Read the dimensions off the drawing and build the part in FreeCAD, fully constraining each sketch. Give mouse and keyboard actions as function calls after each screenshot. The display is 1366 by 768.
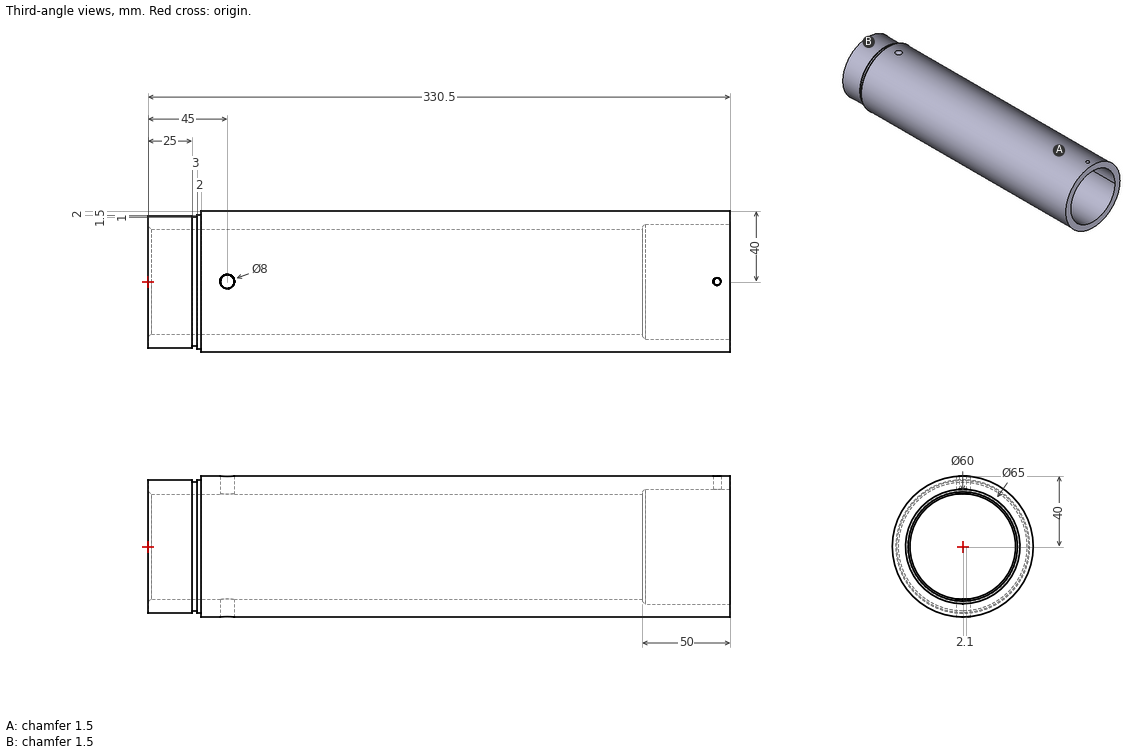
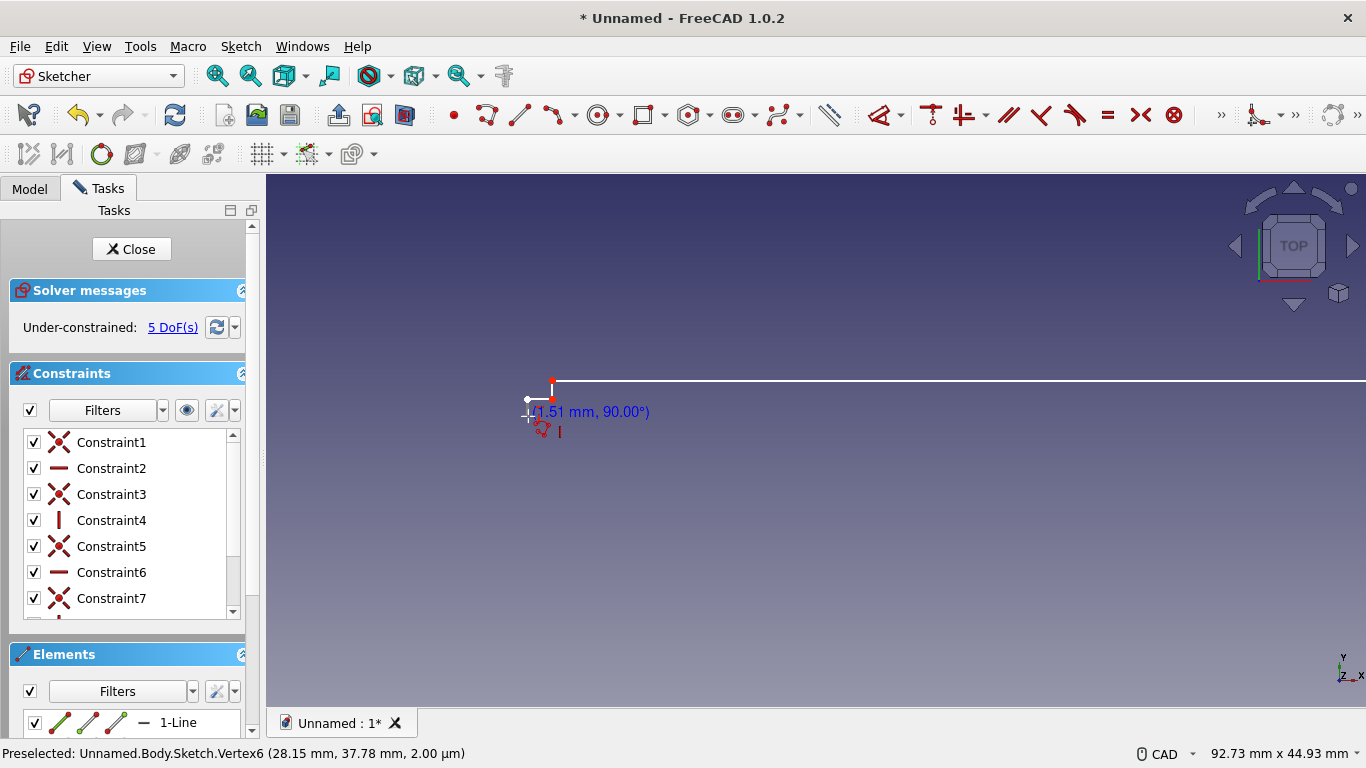
click(528, 416)
click(492, 416)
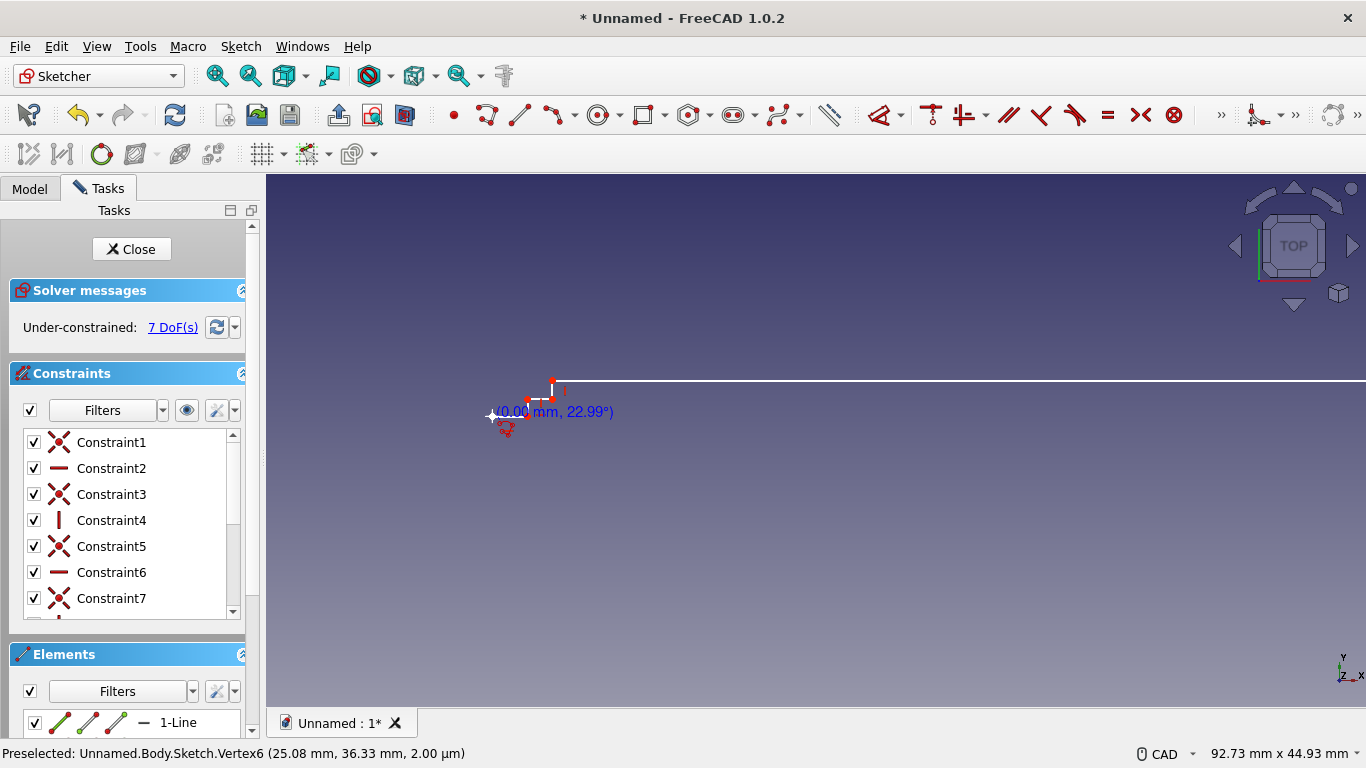
scroll(492, 404, up, 2)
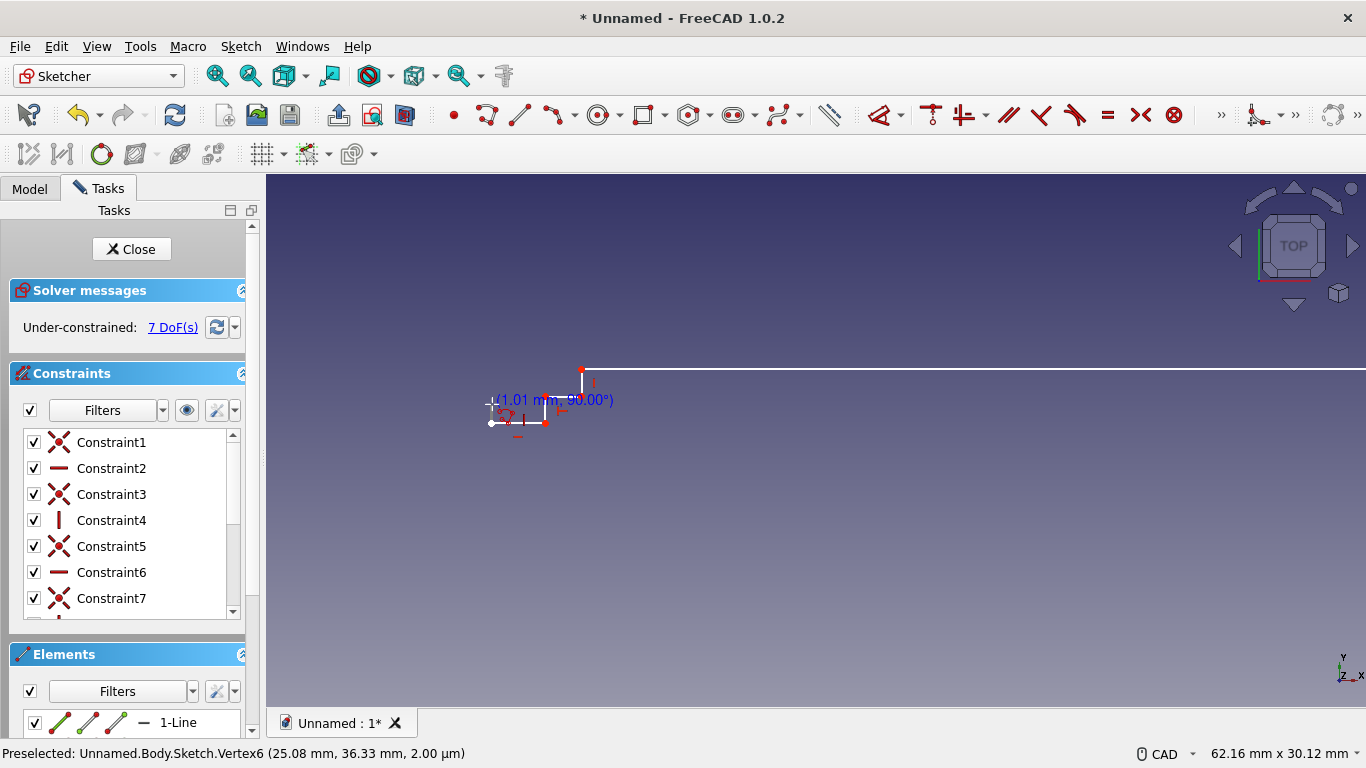
click(492, 404)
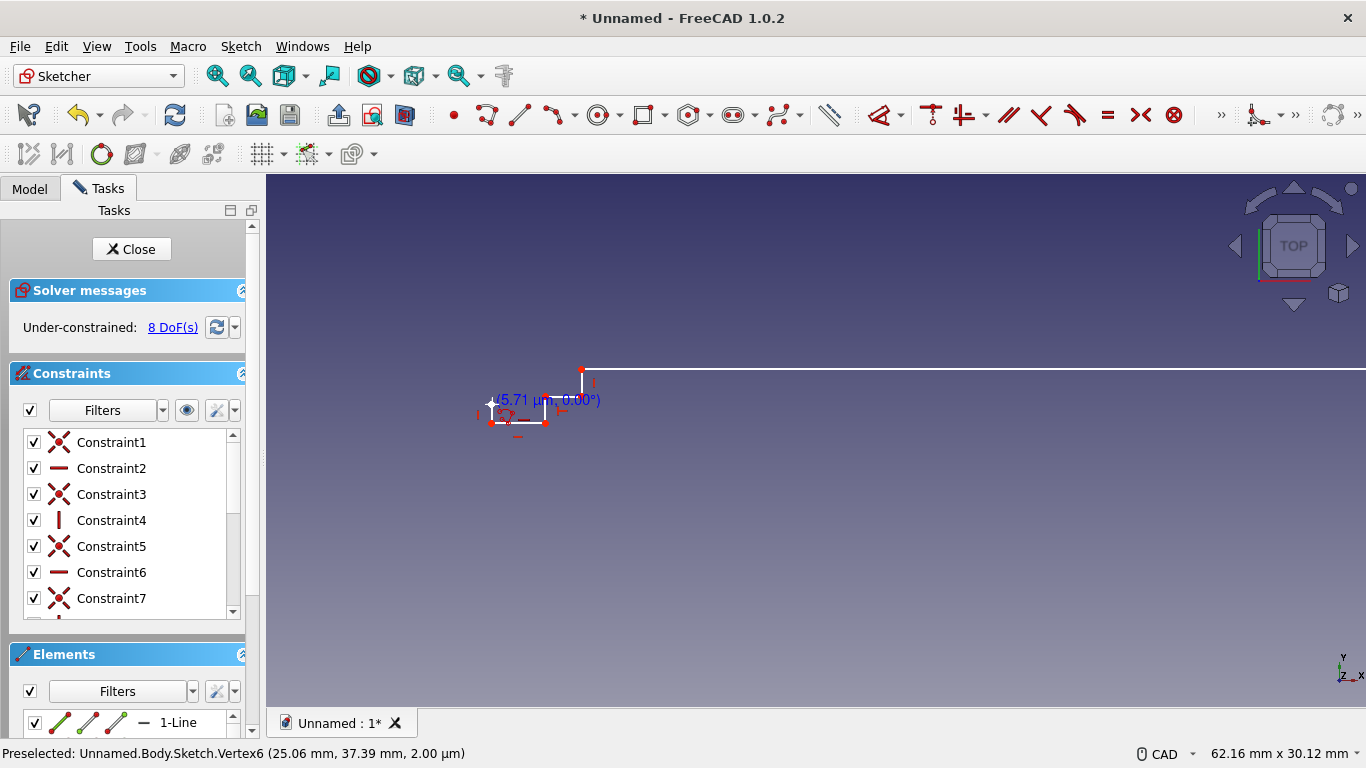
scroll(470, 406, down, 11)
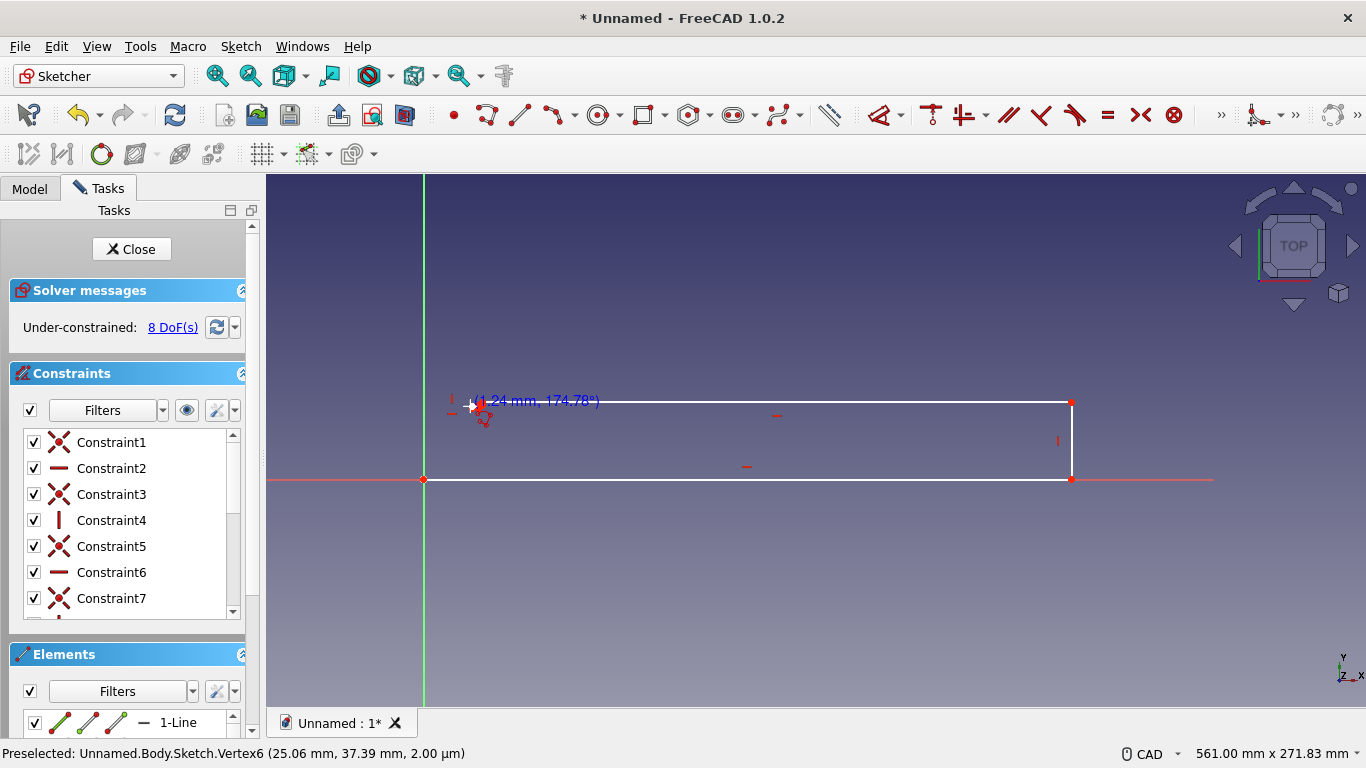
click(433, 406)
click(424, 480)
key(Escape)
key(Escape)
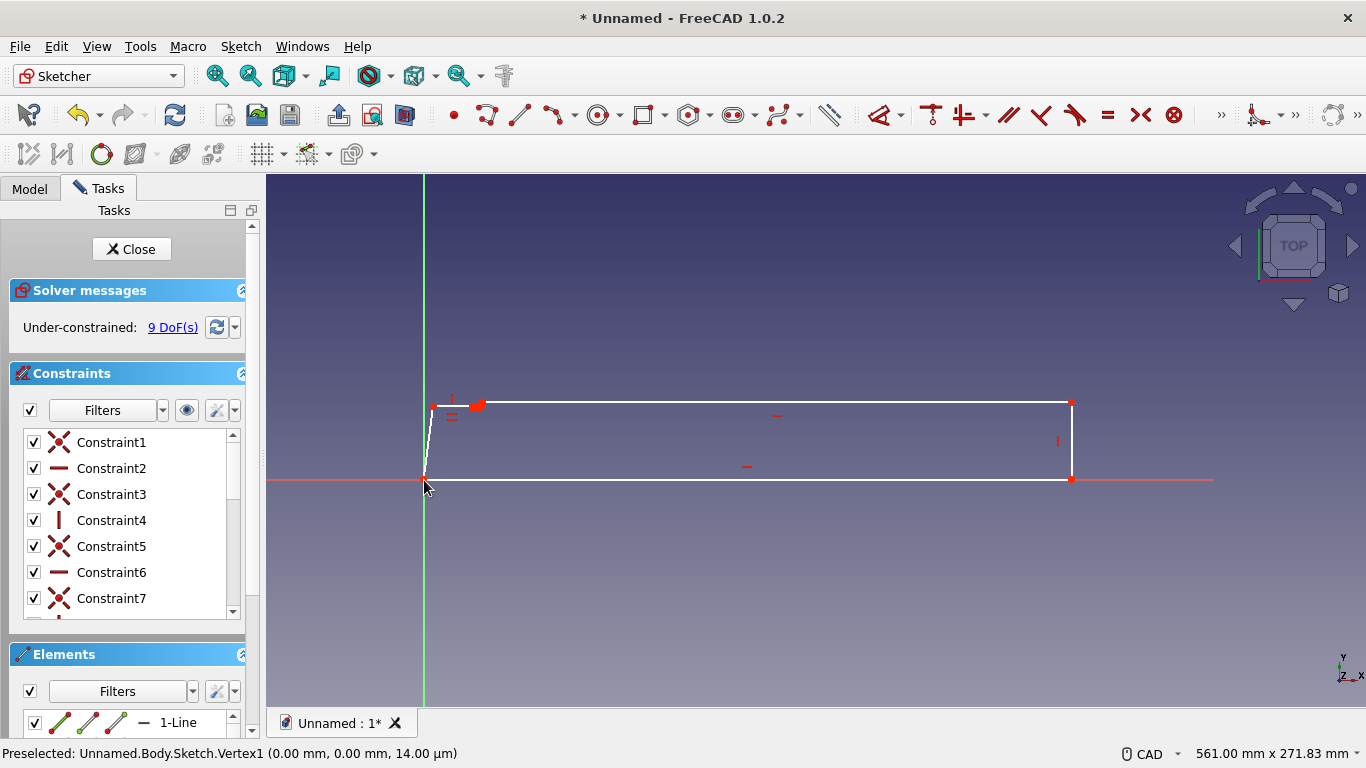
click(426, 458)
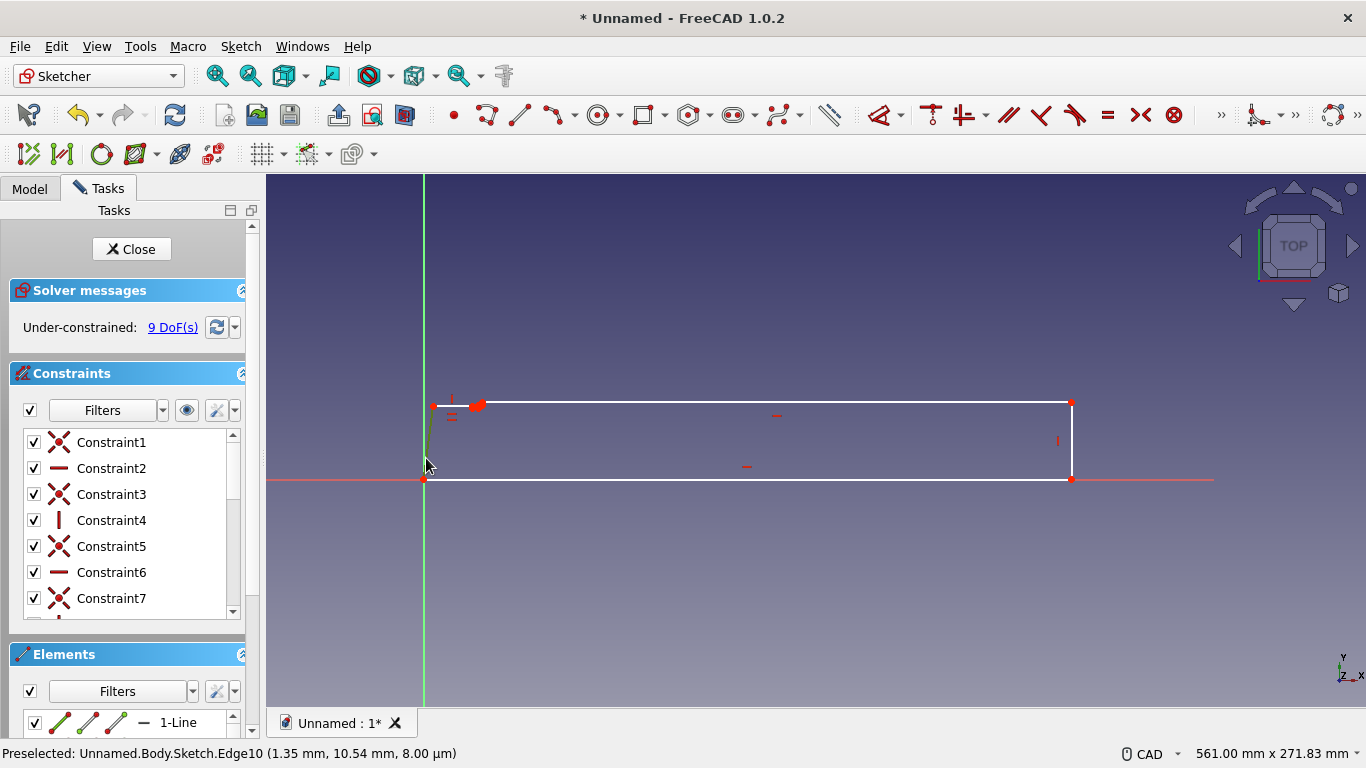
key(v)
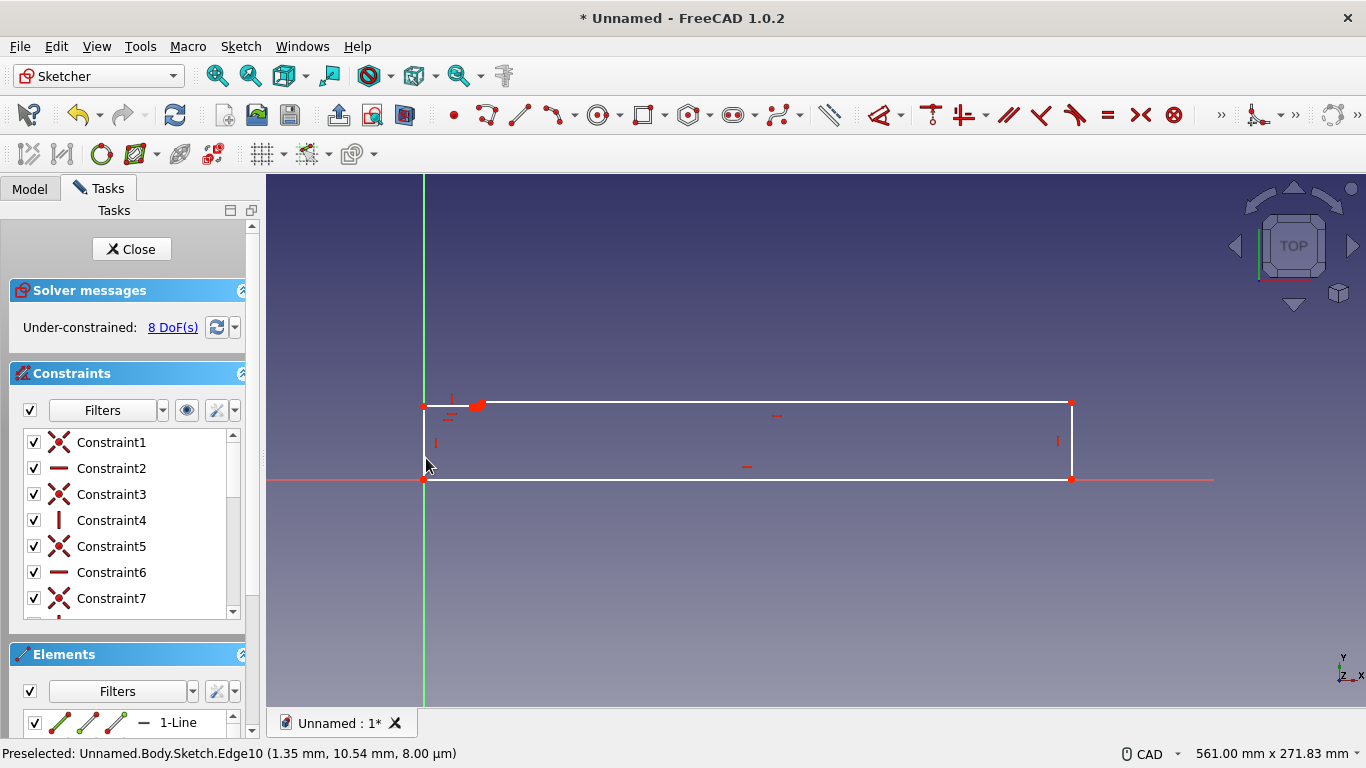
scroll(483, 404, up, 12)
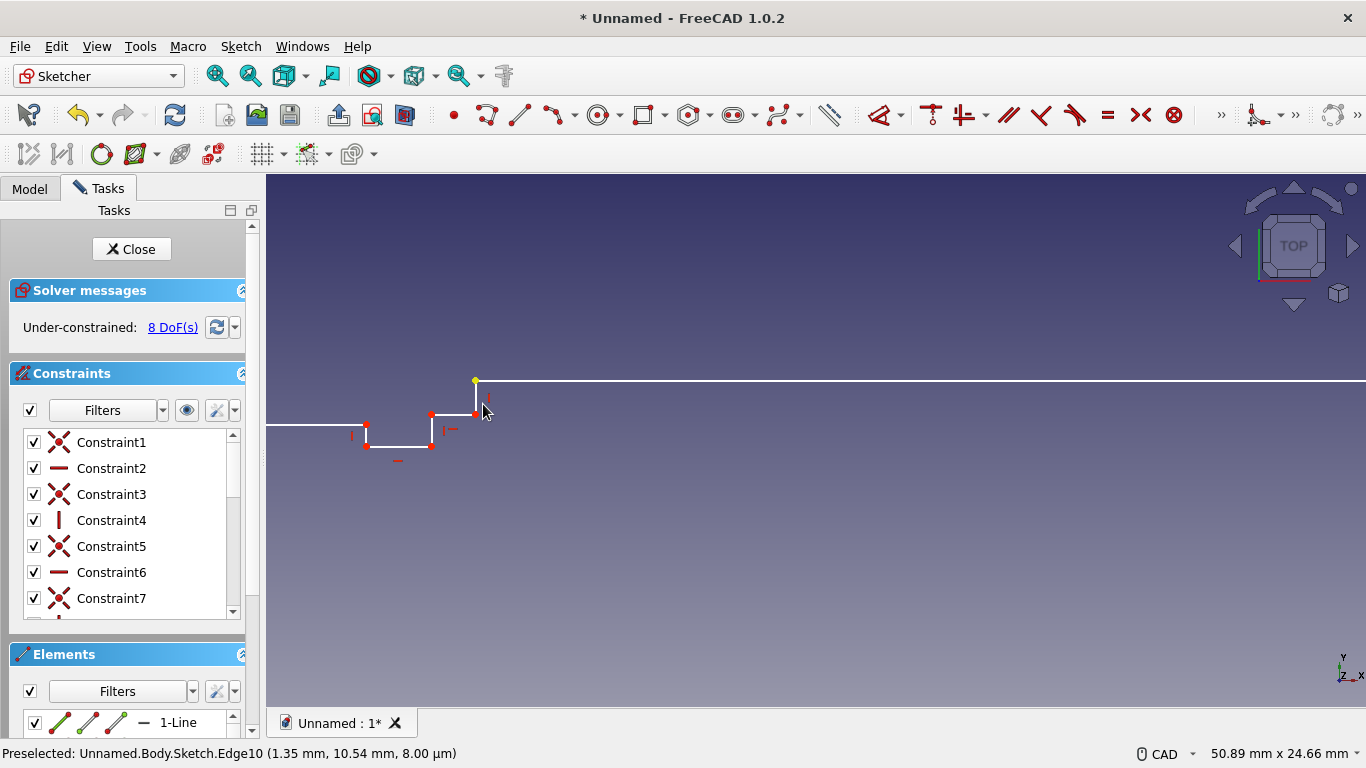
click(476, 398)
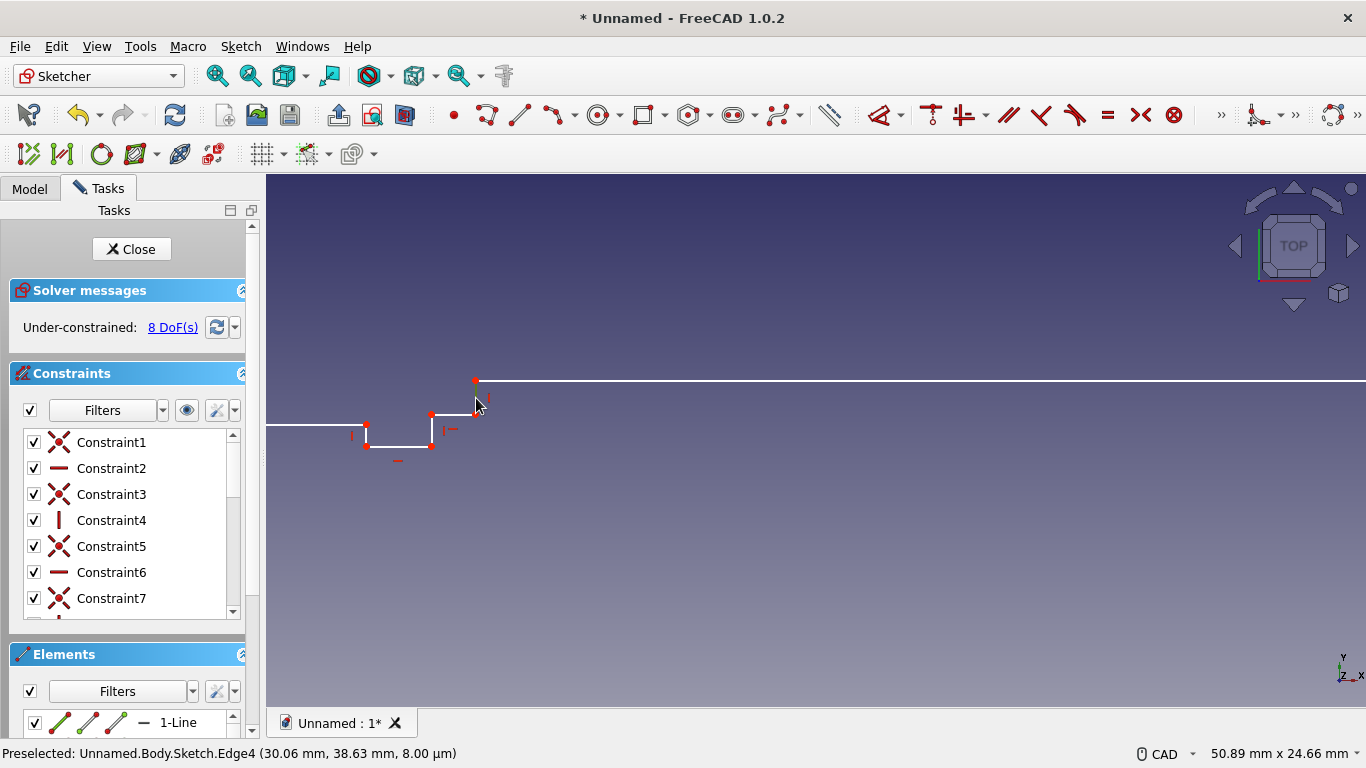
key(i)